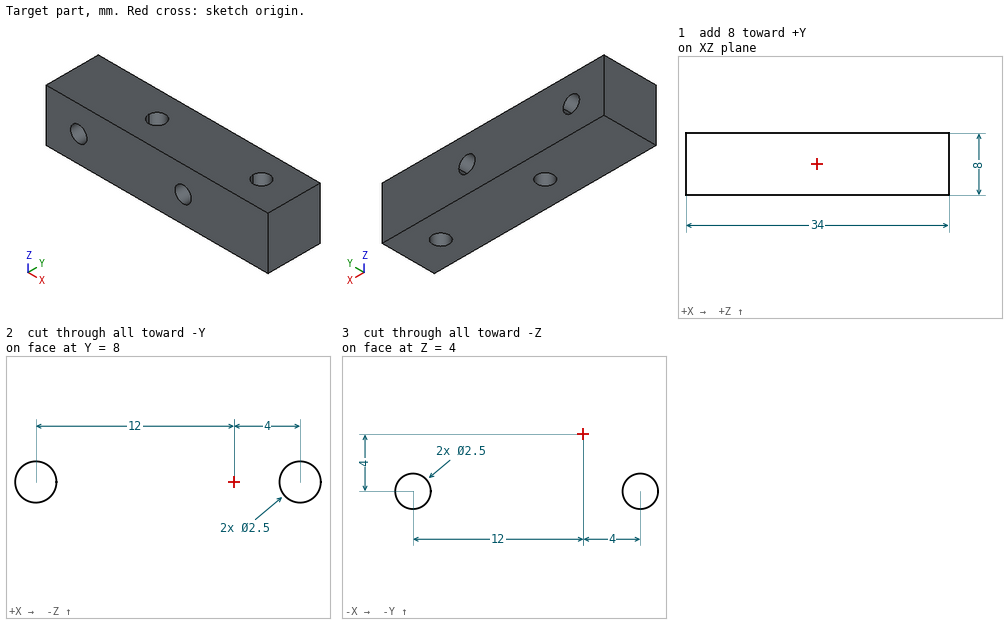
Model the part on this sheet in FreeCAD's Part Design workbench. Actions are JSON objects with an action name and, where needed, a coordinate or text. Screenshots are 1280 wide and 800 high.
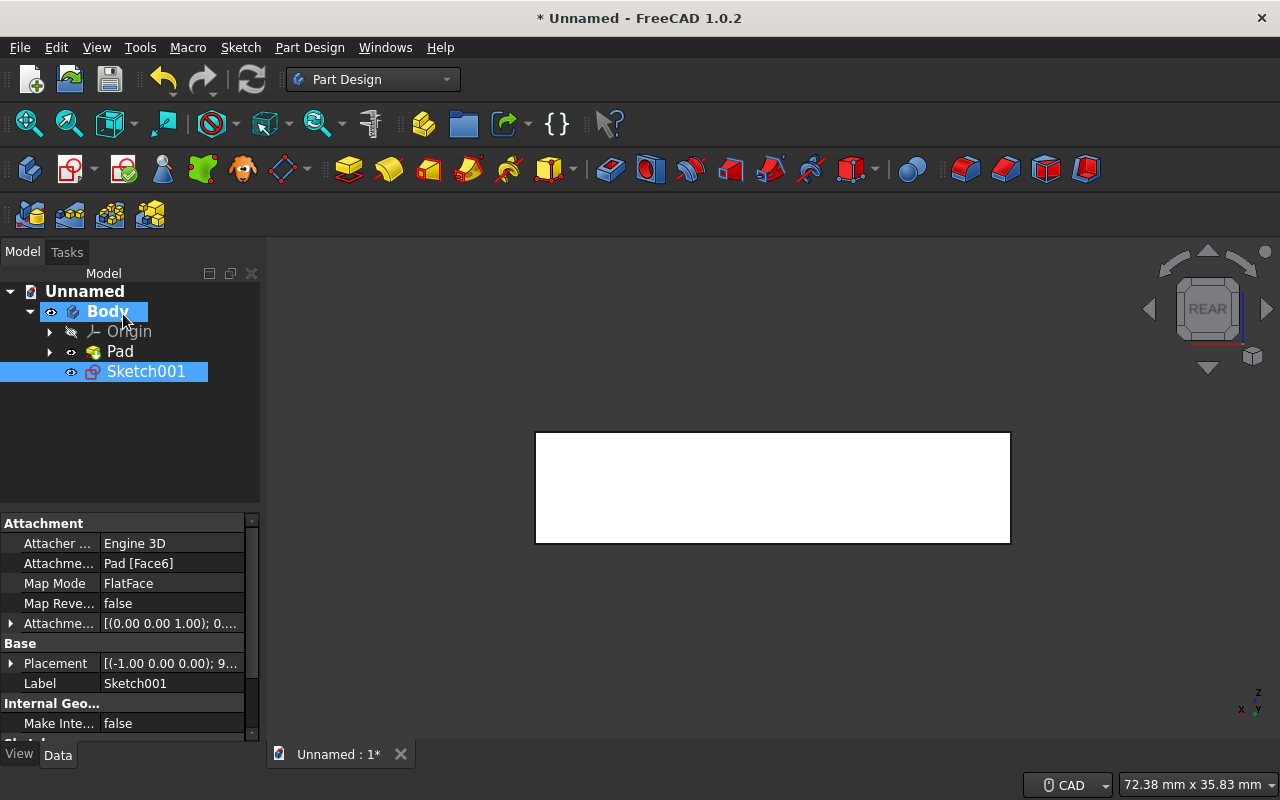
{"action": "left_click", "coordinate": [612, 170]}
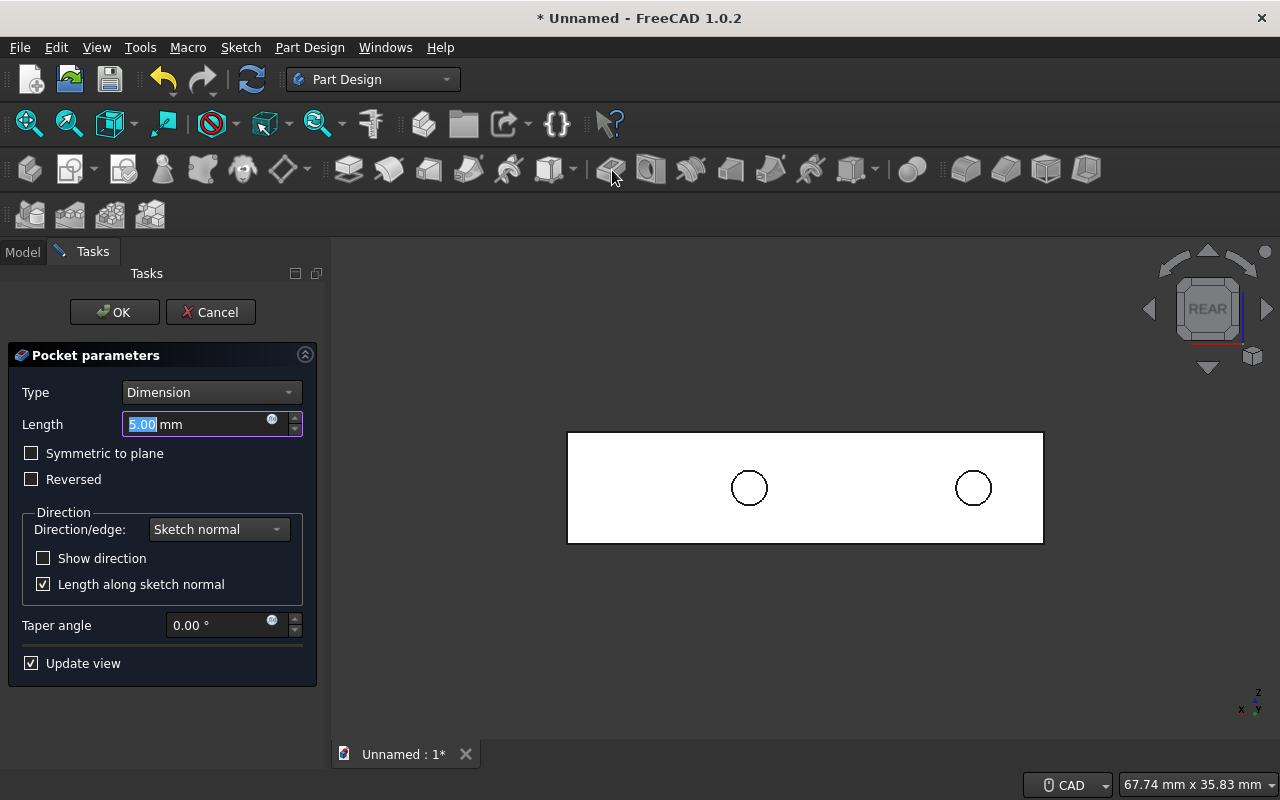
{"action": "left_click", "coordinate": [212, 392]}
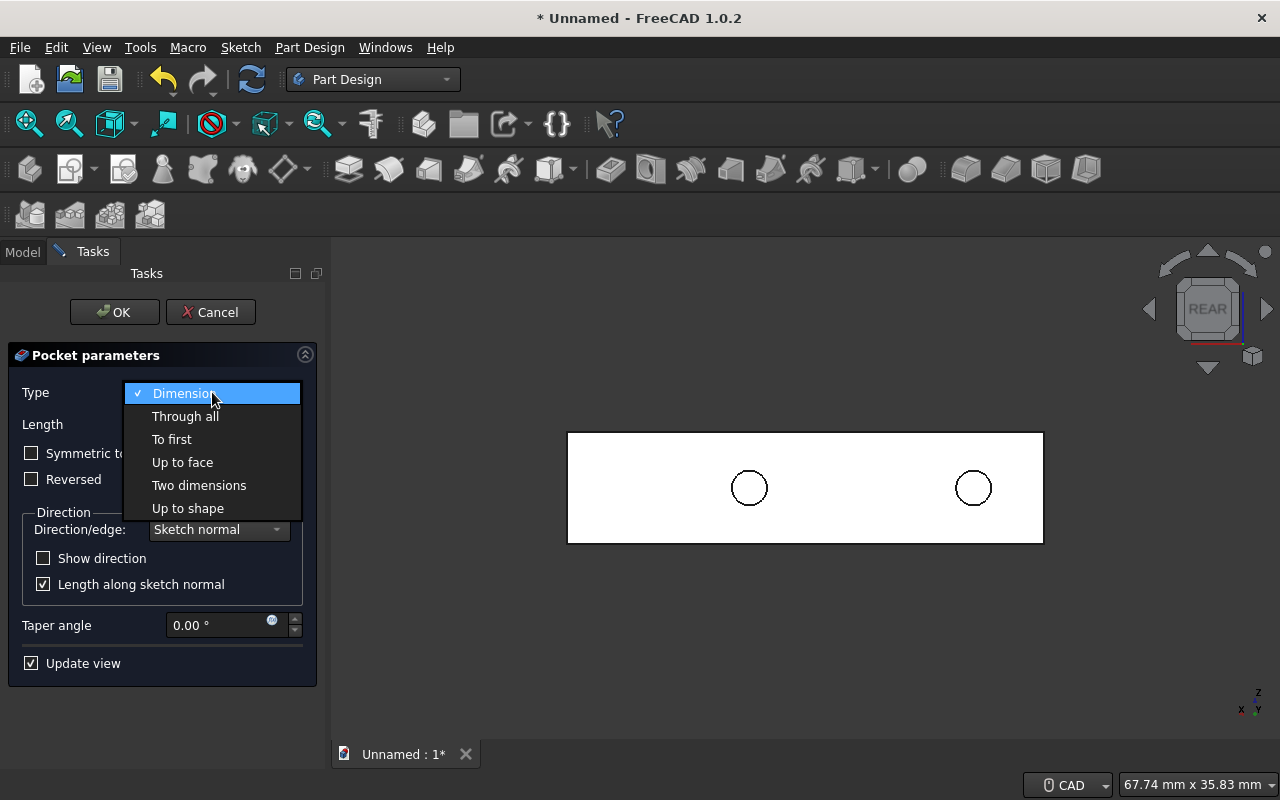
{"action": "left_click", "coordinate": [212, 416]}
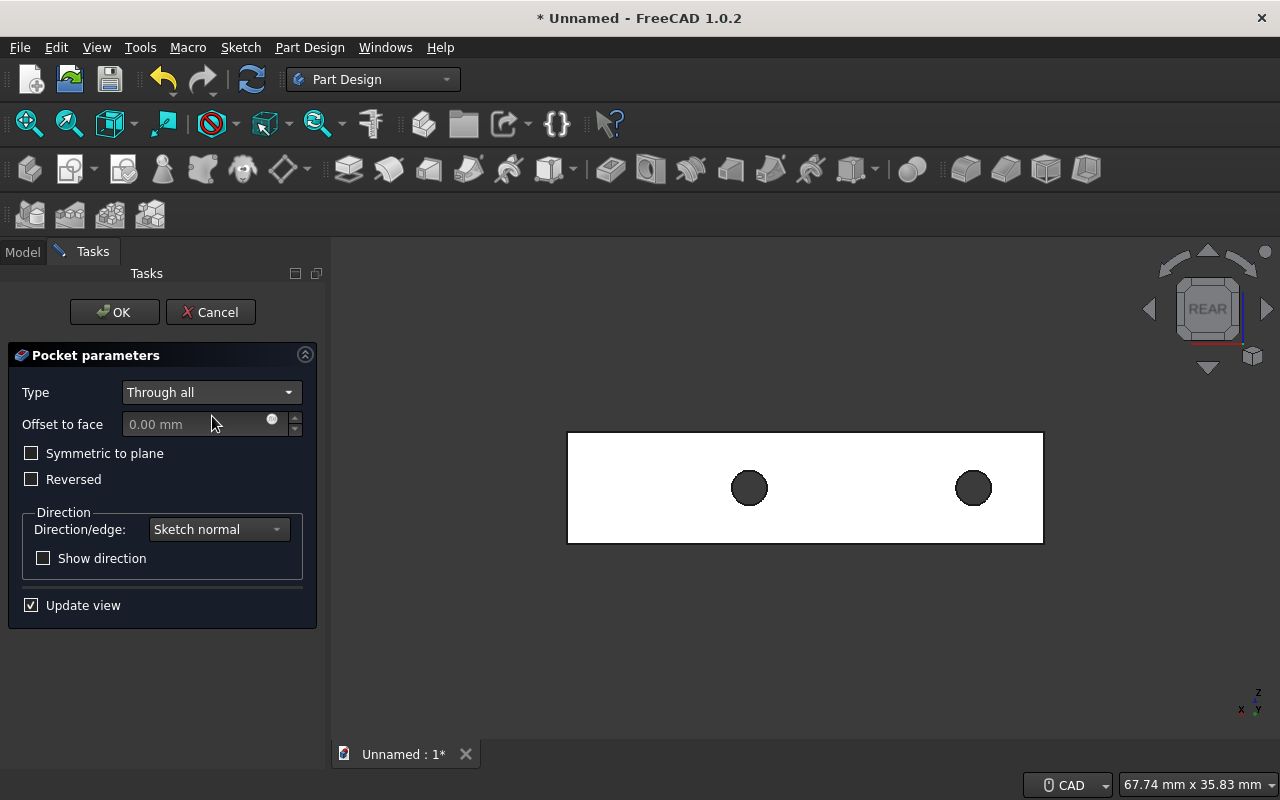
{"action": "left_click", "coordinate": [115, 312]}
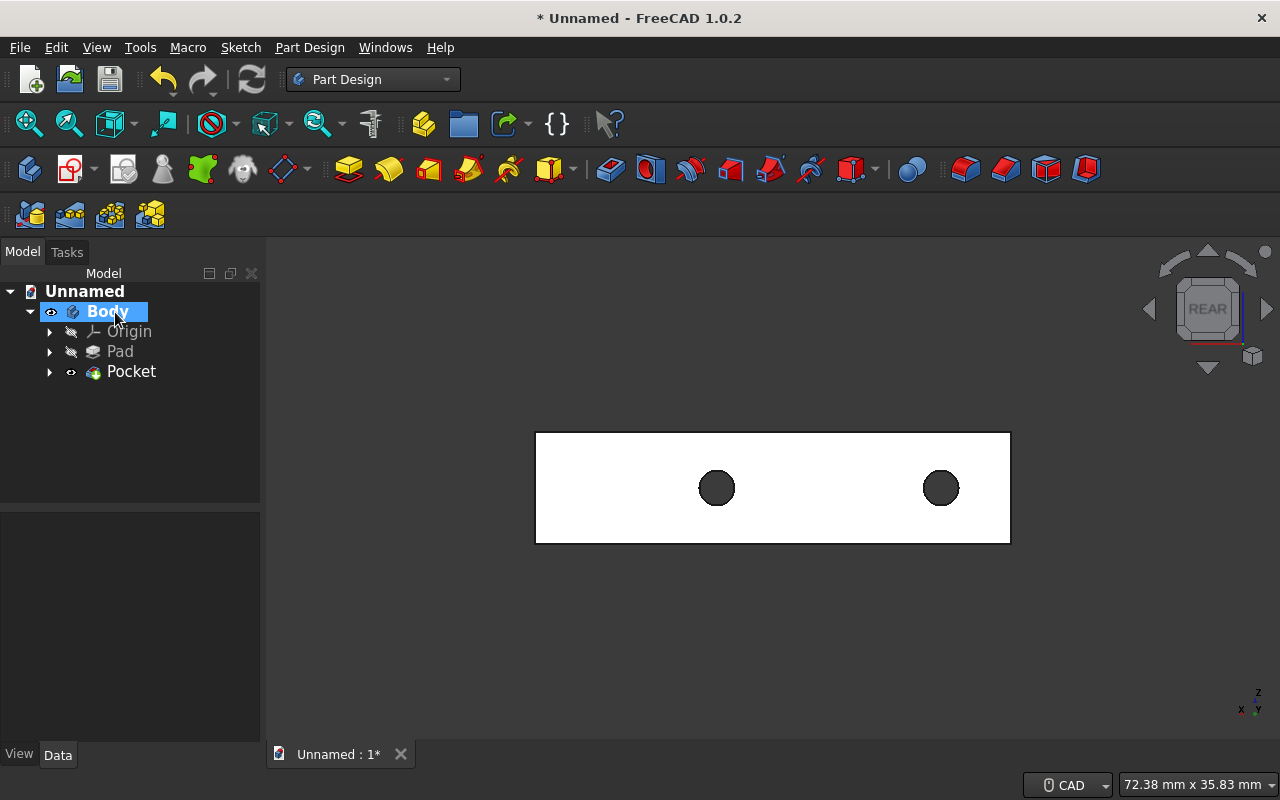
{"action": "key", "text": "0"}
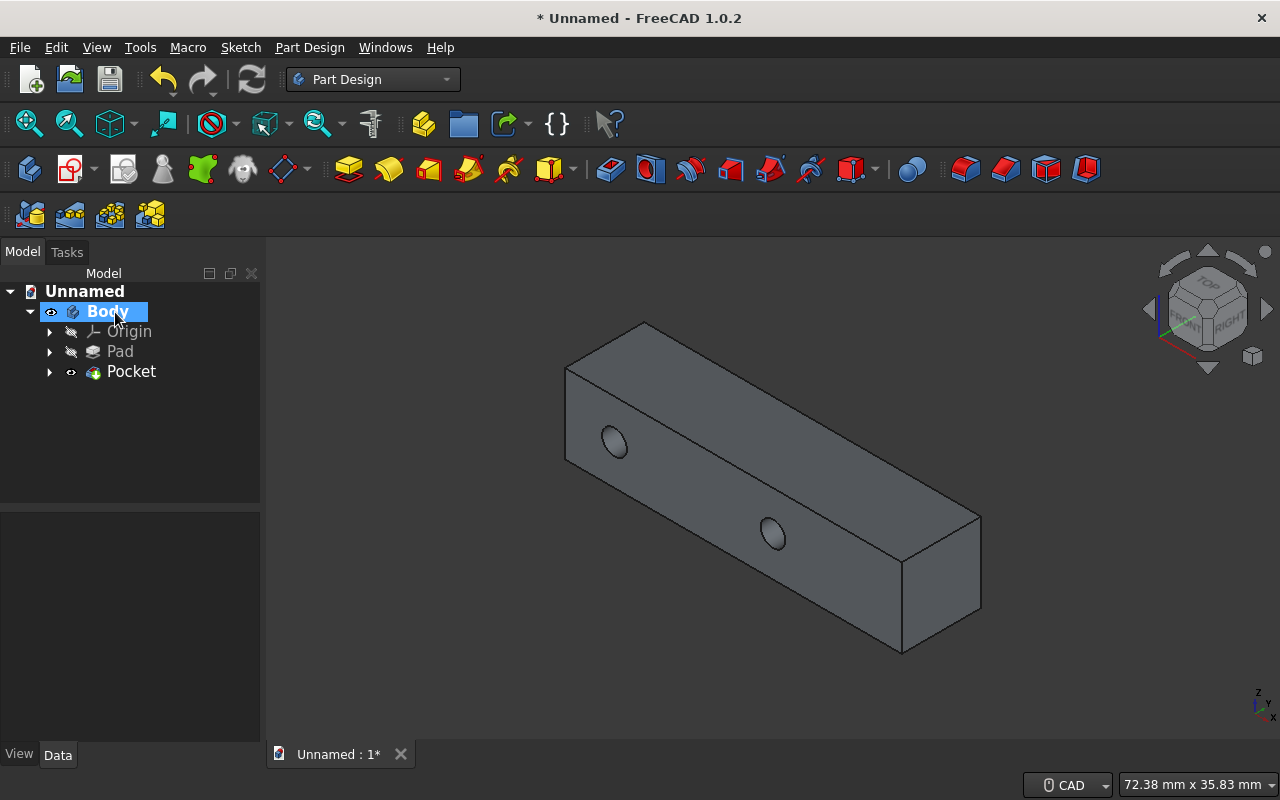
{"action": "left_click", "coordinate": [869, 497]}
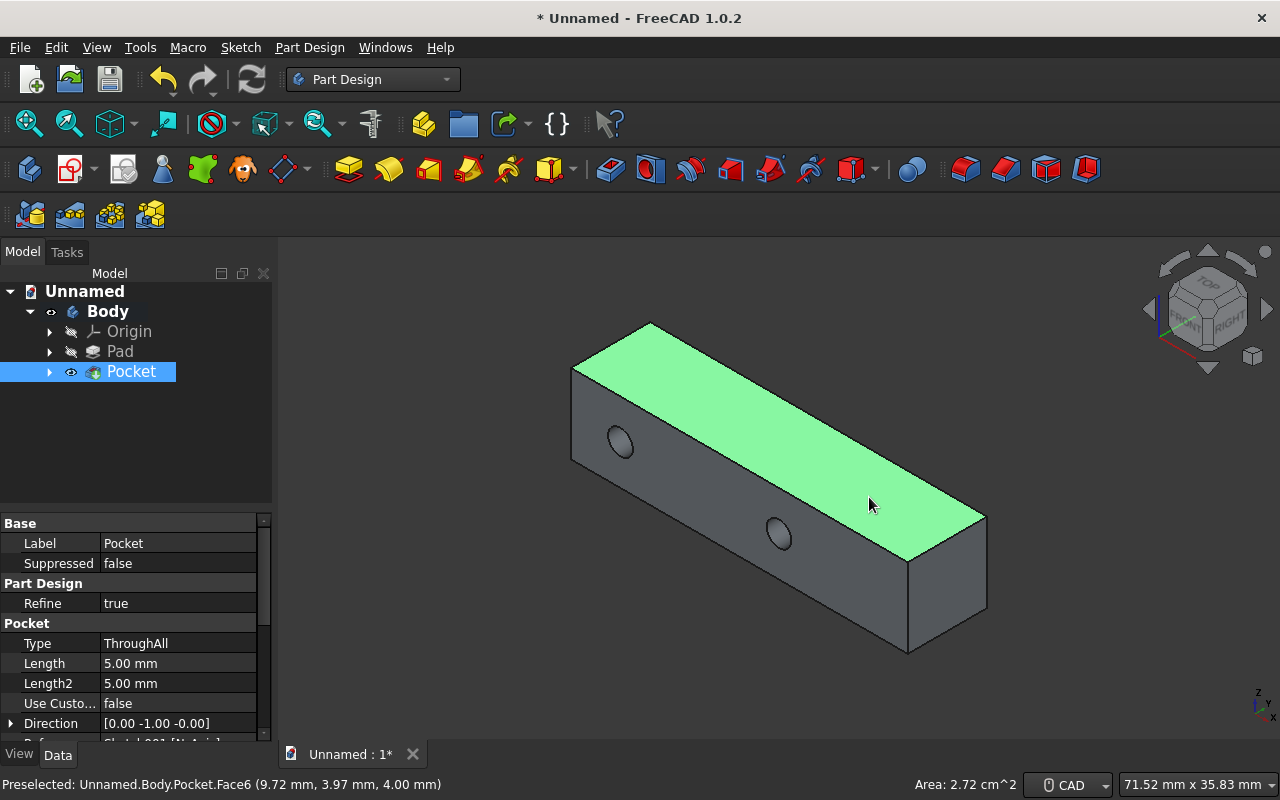
{"action": "left_click", "coordinate": [70, 170]}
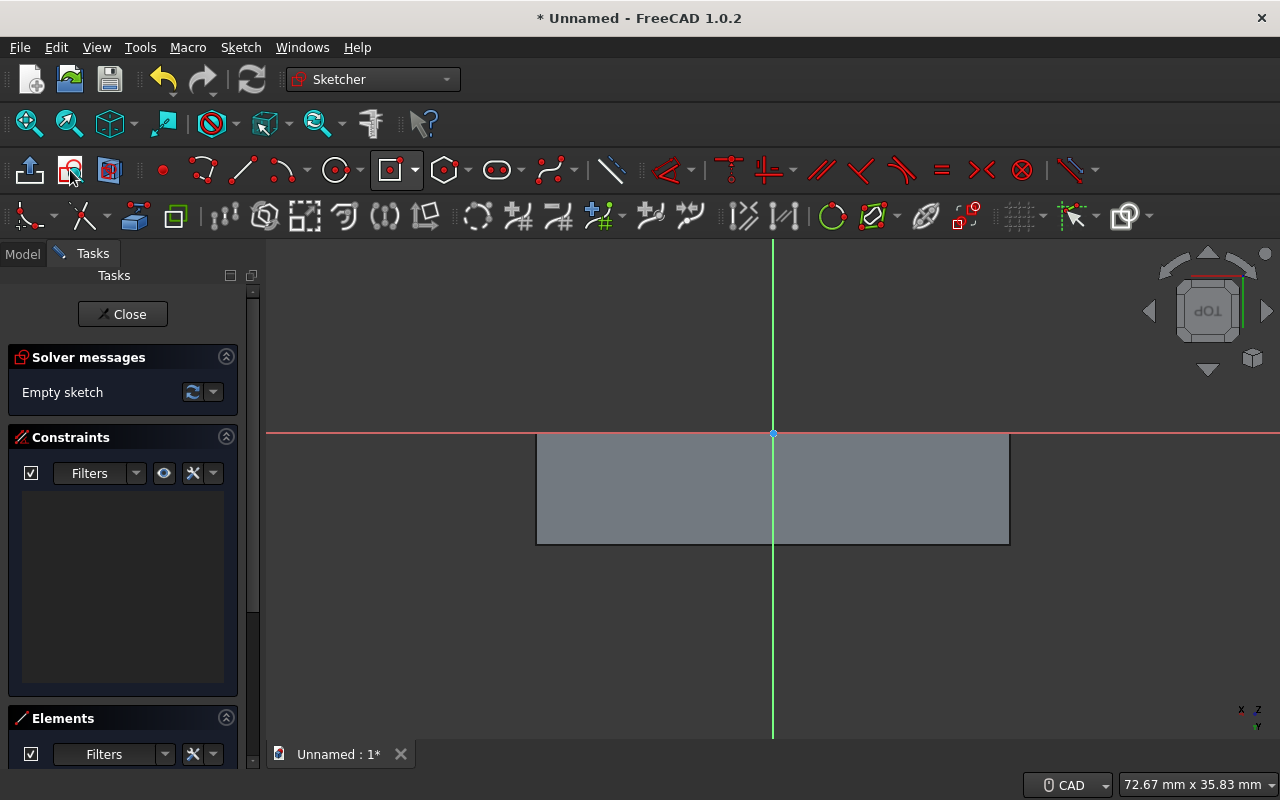
{"action": "scroll", "coordinate": [728, 454], "scroll_direction": "up", "scroll_amount": 4}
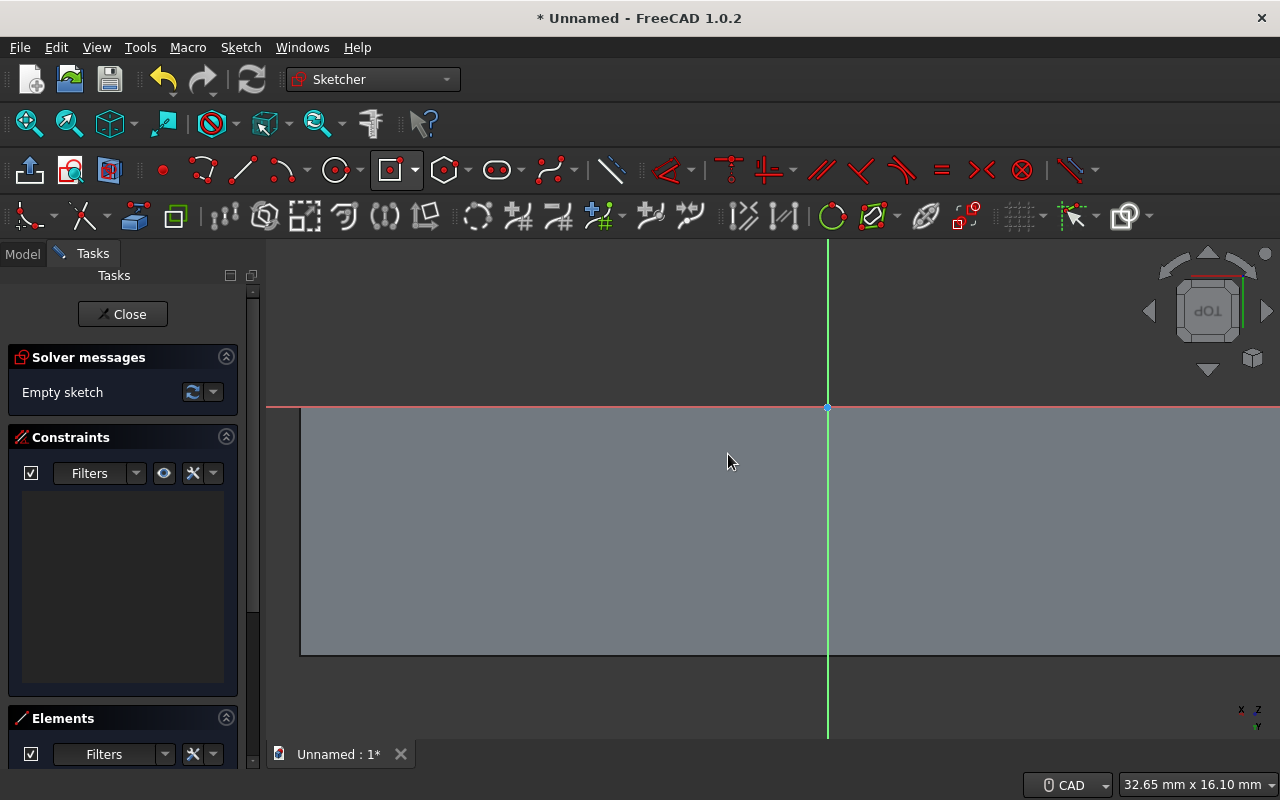
{"action": "left_click", "coordinate": [336, 170]}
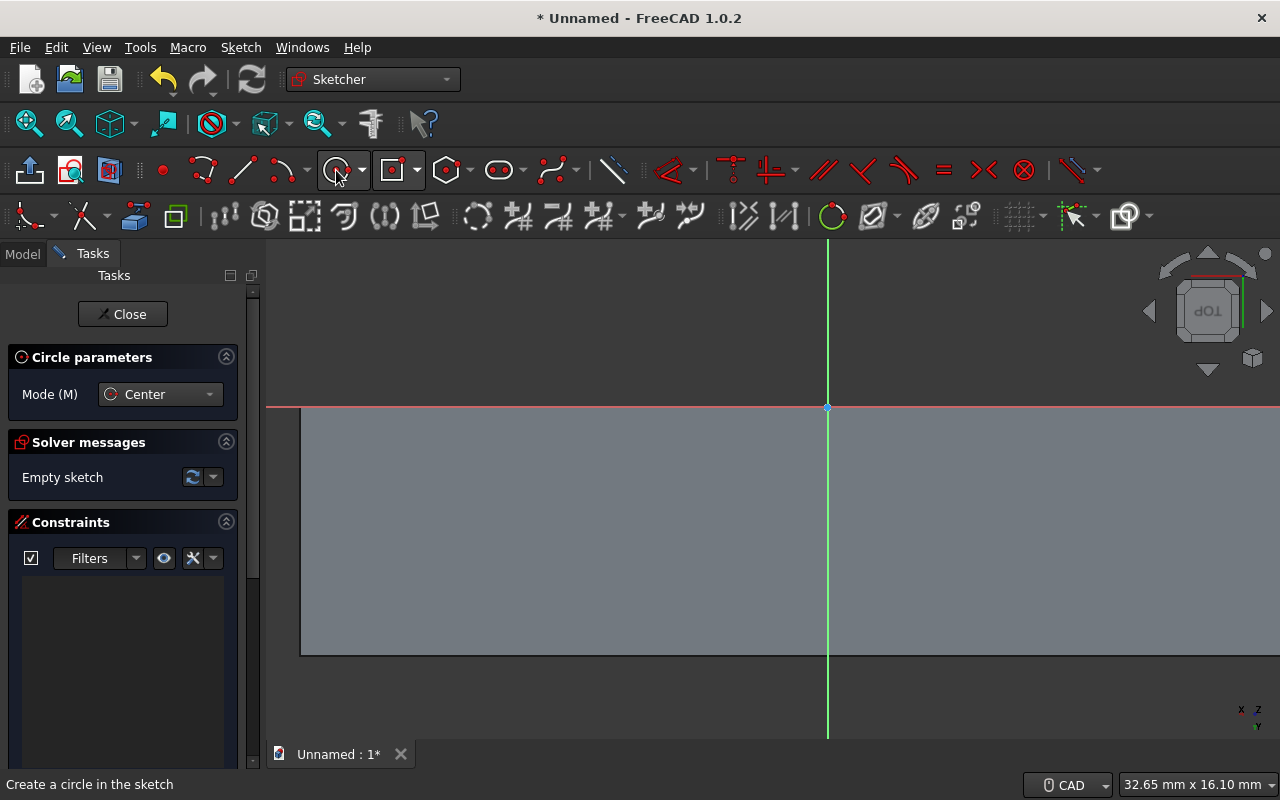
{"action": "left_click", "coordinate": [455, 531]}
{"action": "mouse_move", "coordinate": [482, 504]}